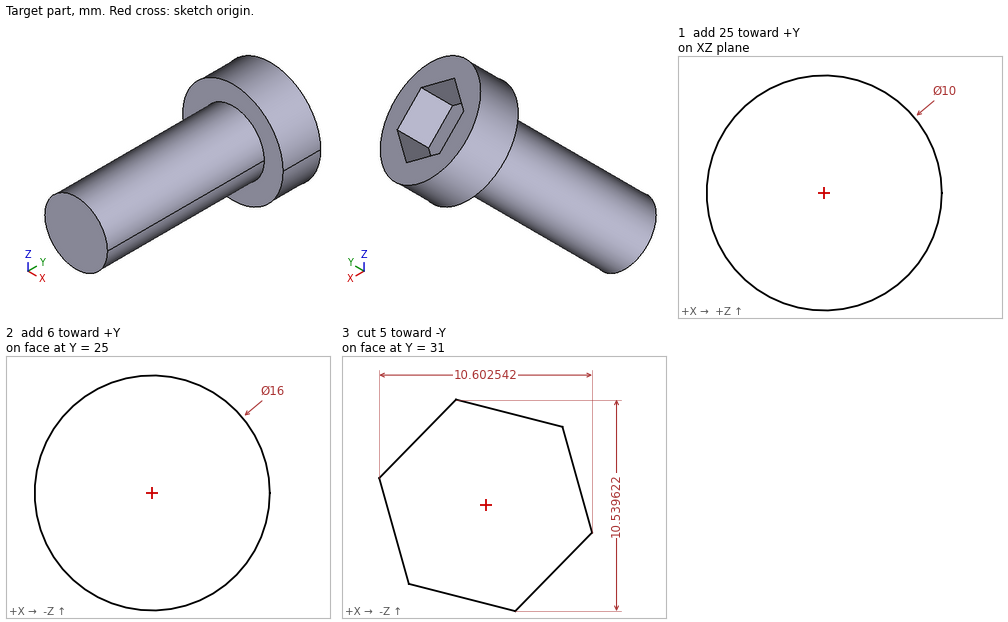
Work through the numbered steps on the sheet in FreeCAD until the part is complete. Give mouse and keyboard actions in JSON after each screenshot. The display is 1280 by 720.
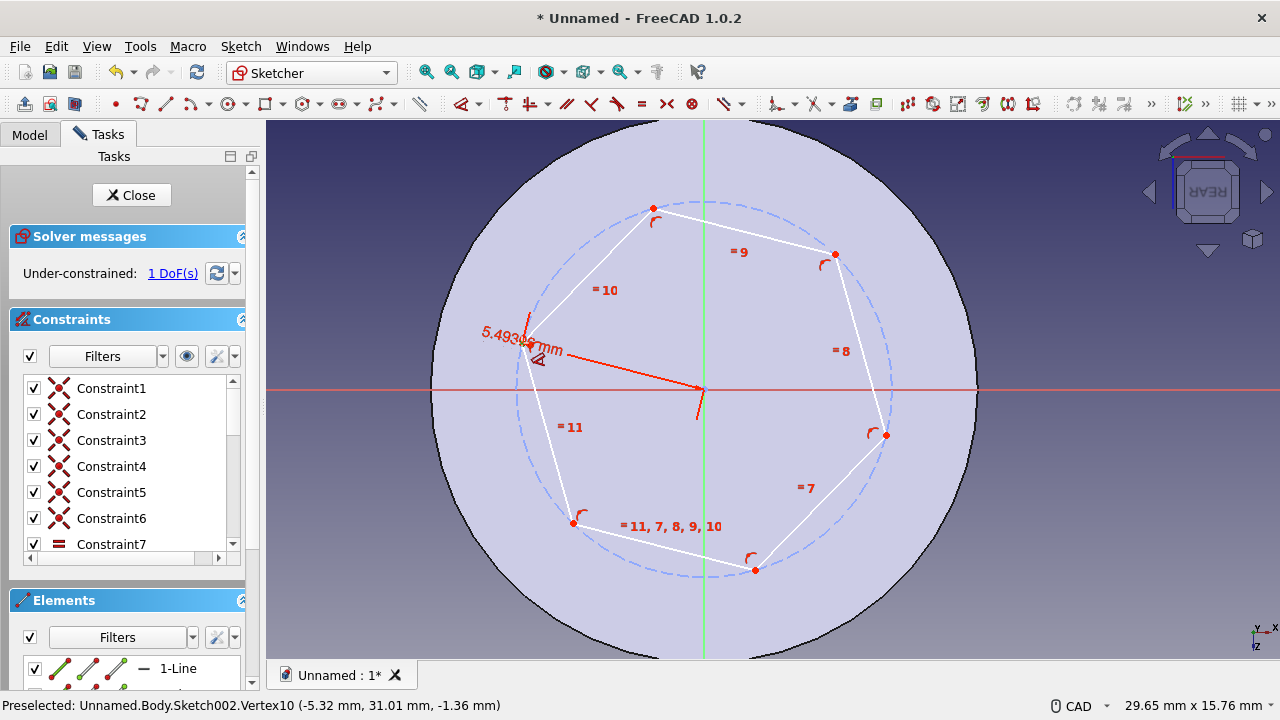
{"action": "left_click", "coordinate": [886, 436]}
{"action": "left_click", "coordinate": [620, 309]}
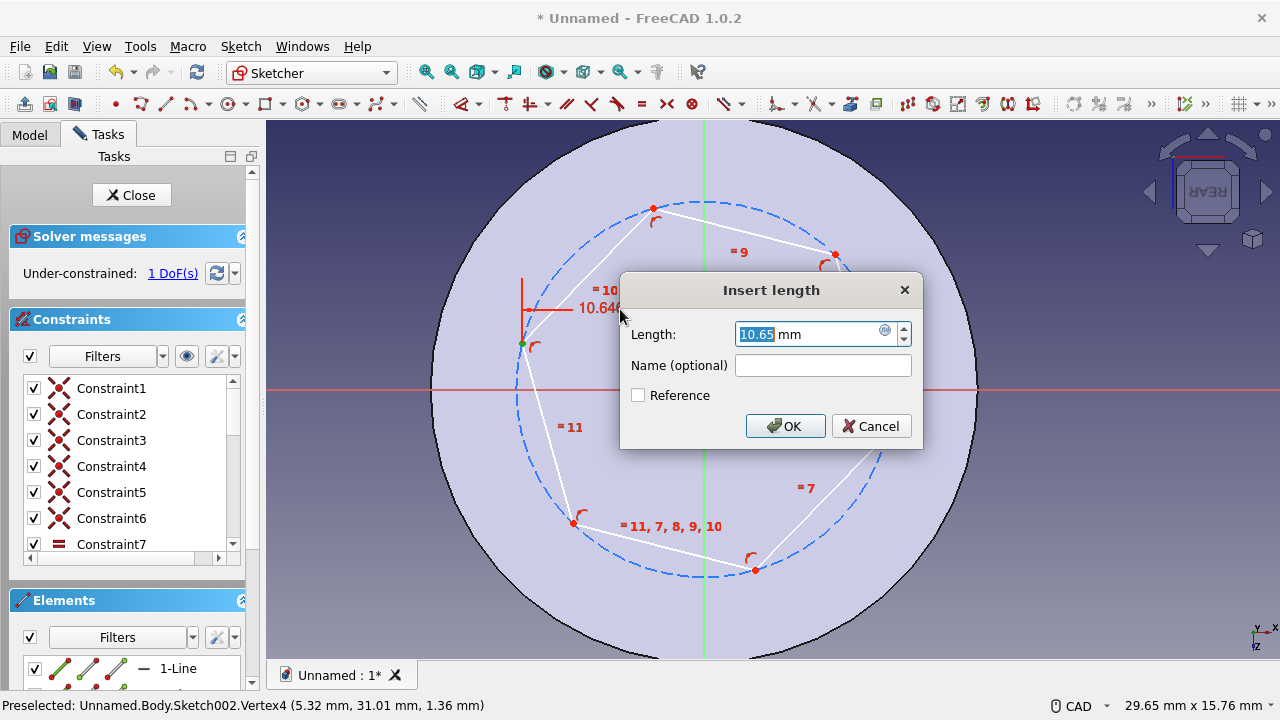
{"action": "type", "text": "10.602542"}
{"action": "key", "text": "Return"}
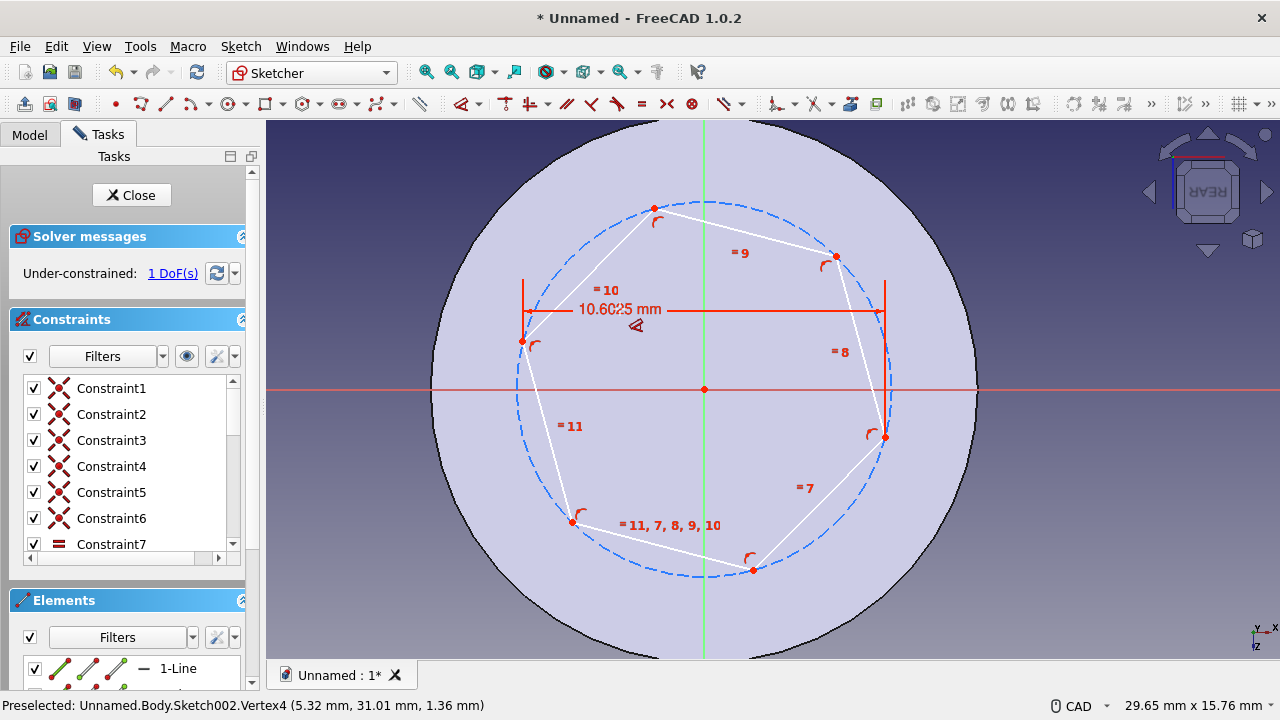
{"action": "left_click", "coordinate": [754, 570]}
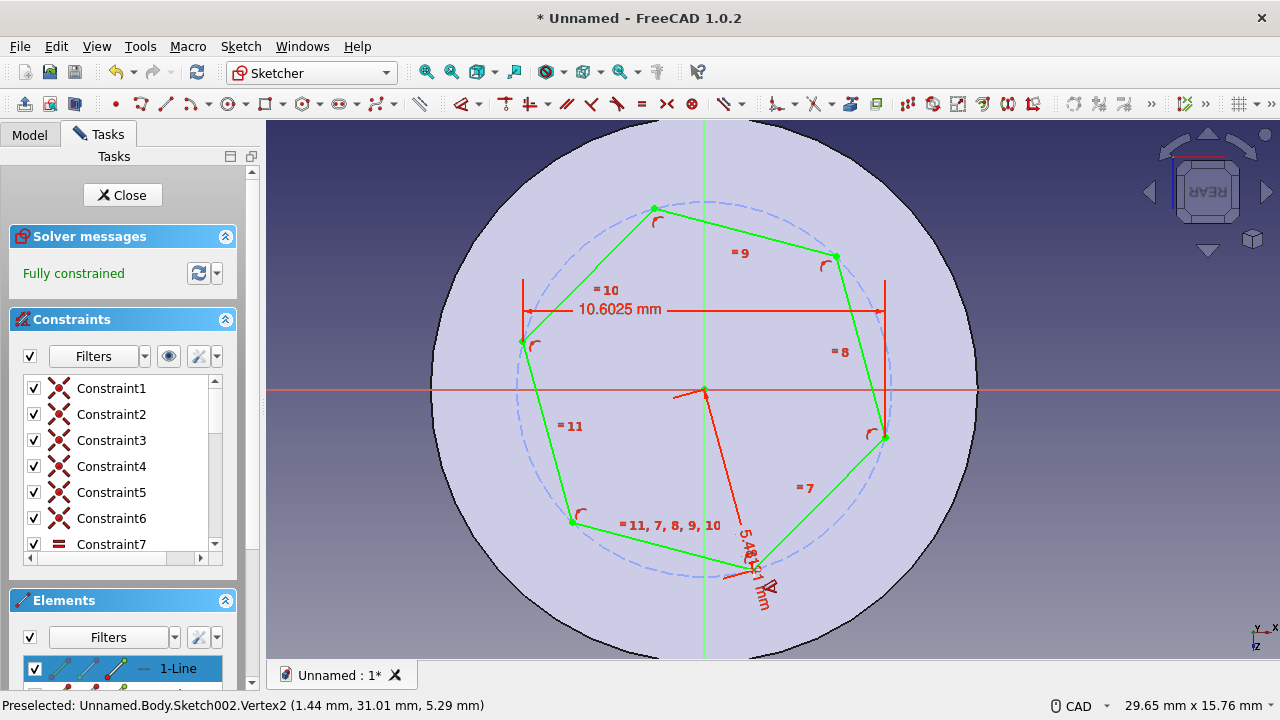
{"action": "left_click", "coordinate": [655, 209]}
{"action": "left_click", "coordinate": [788, 306]}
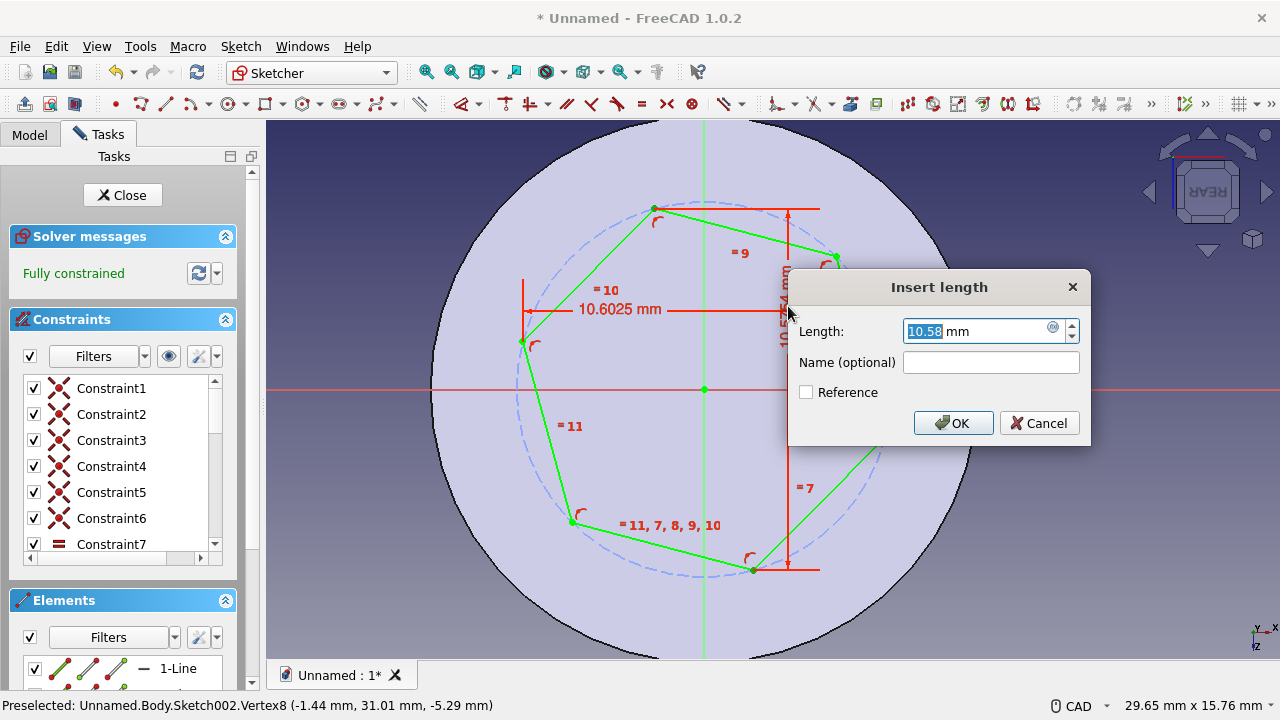
{"action": "type", "text": "10.539622"}
{"action": "key", "text": "Return"}
{"action": "key", "text": "Escape"}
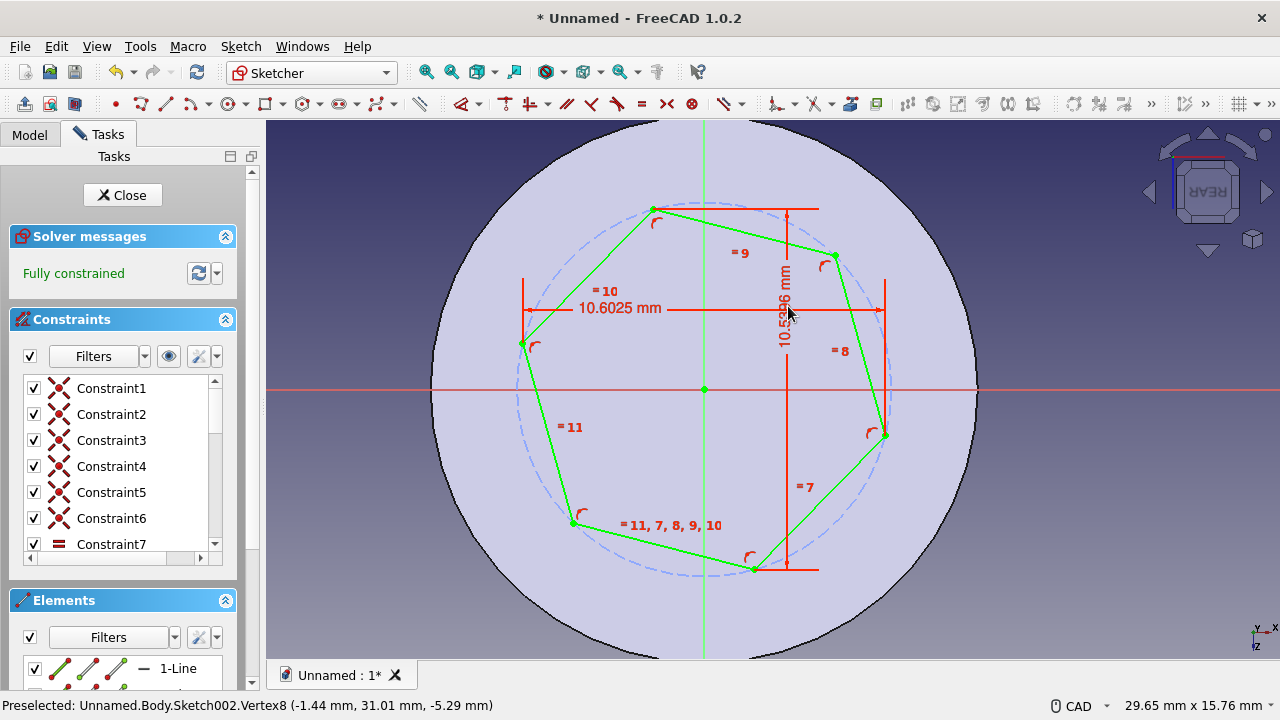
{"action": "left_click", "coordinate": [123, 195]}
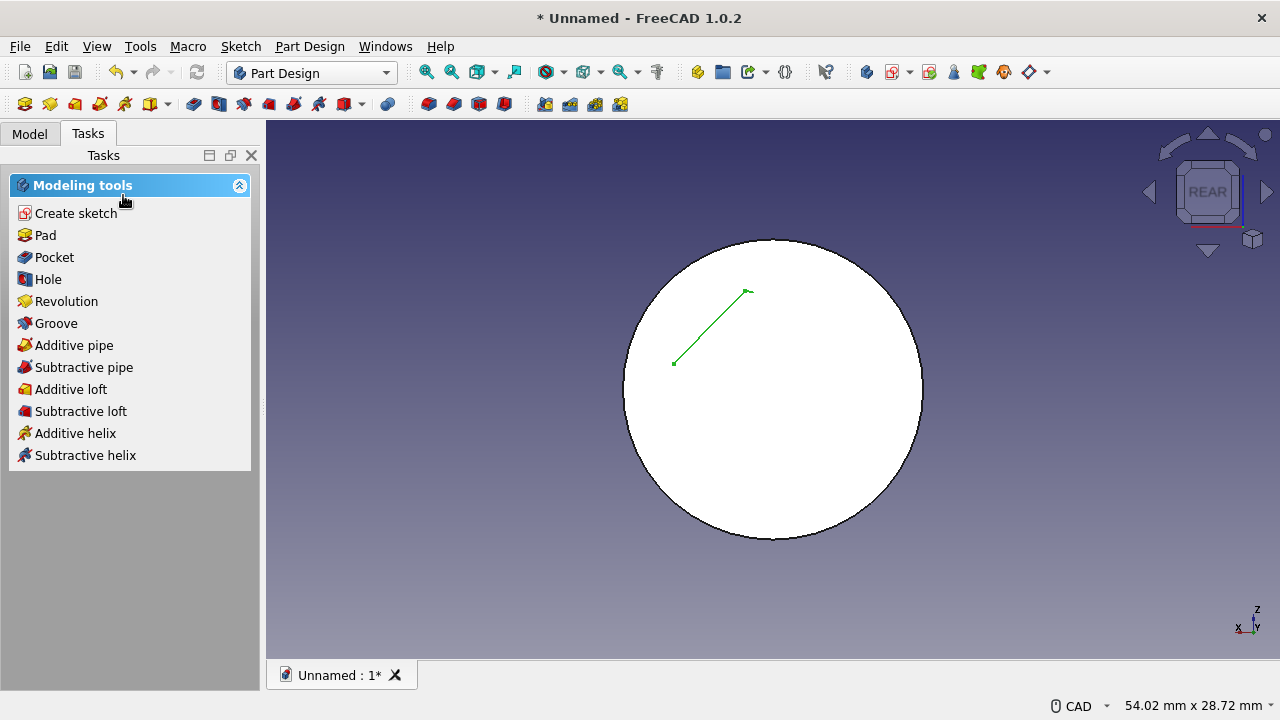
{"action": "left_click", "coordinate": [194, 104]}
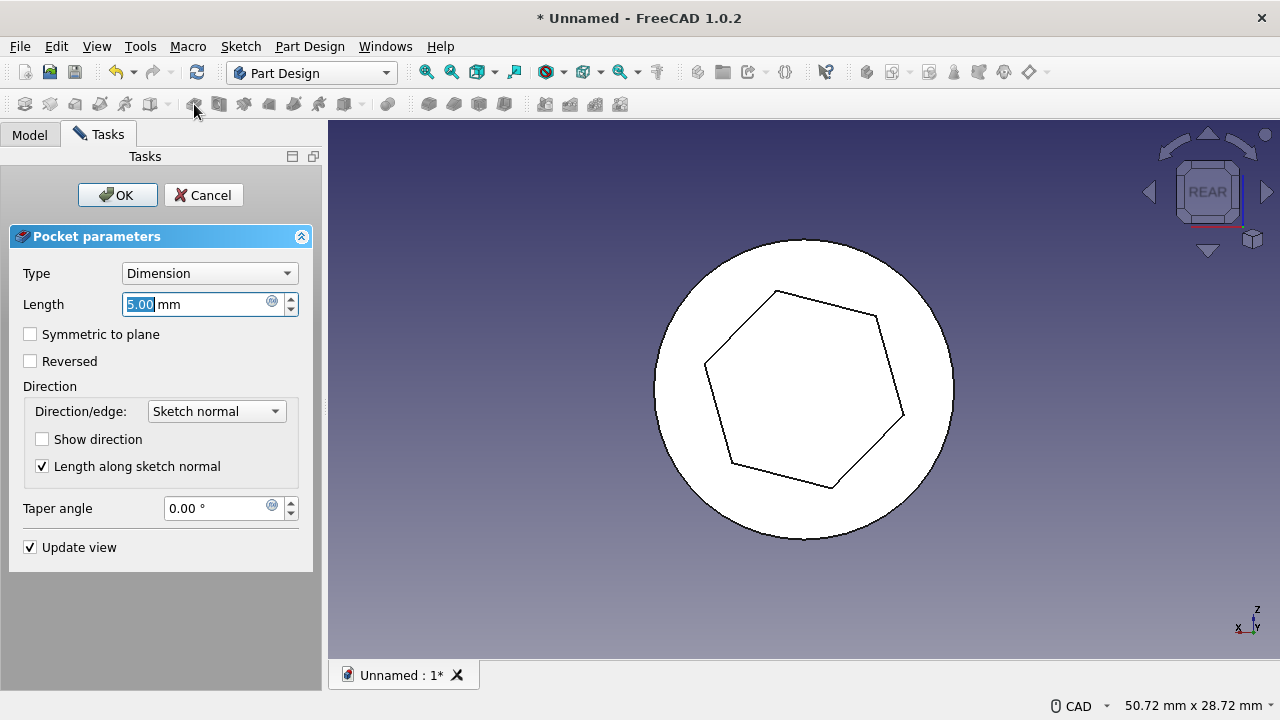
{"action": "type", "text": "5"}
{"action": "key", "text": "Tab"}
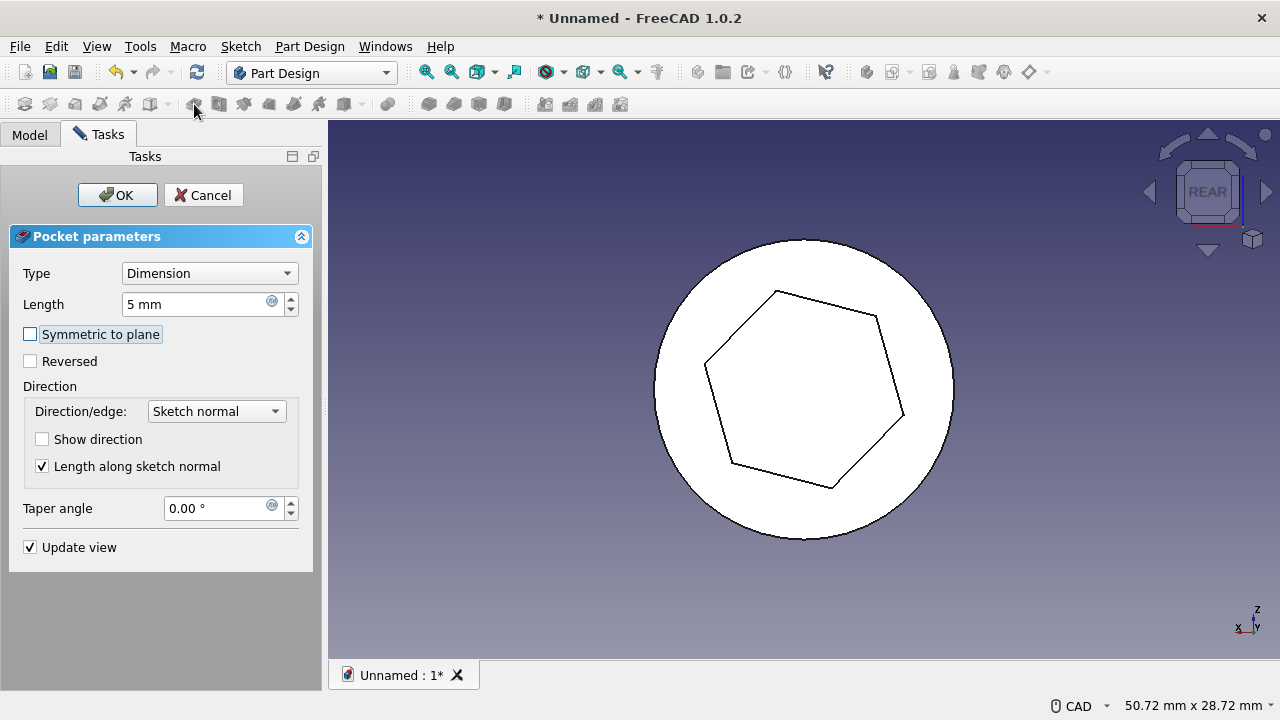
{"action": "left_click", "coordinate": [118, 195]}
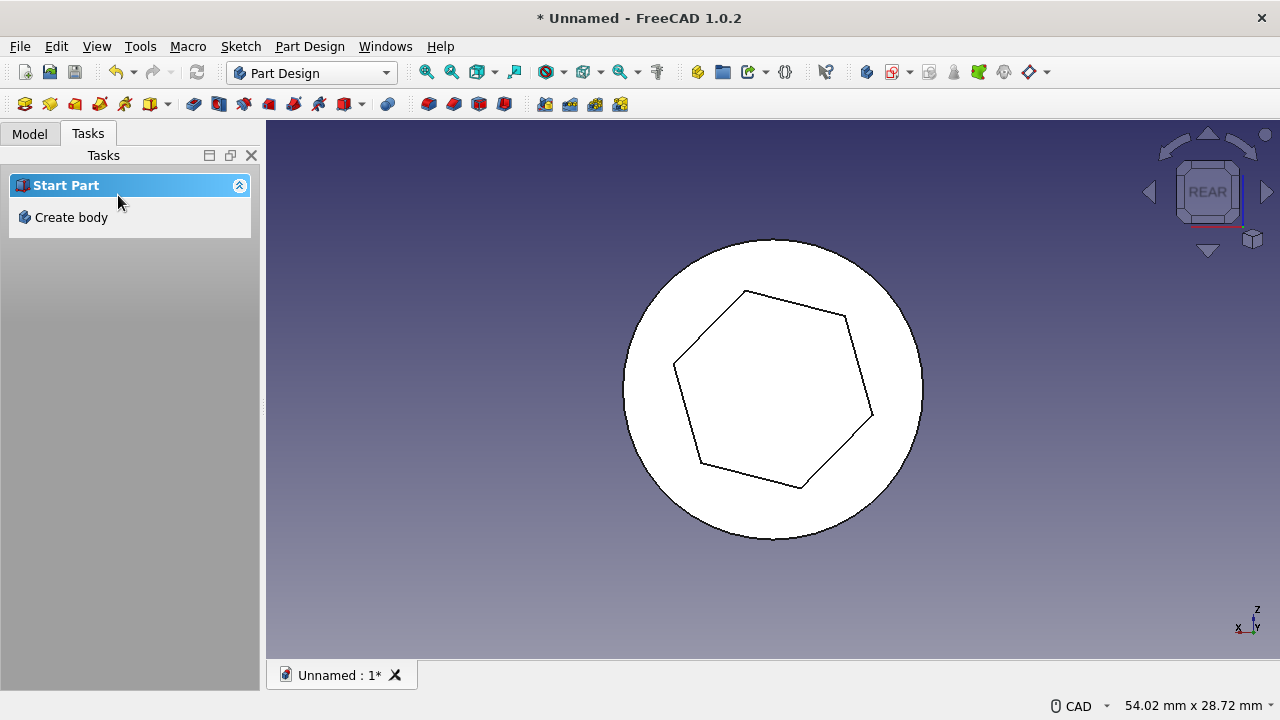
{"action": "key", "text": "0"}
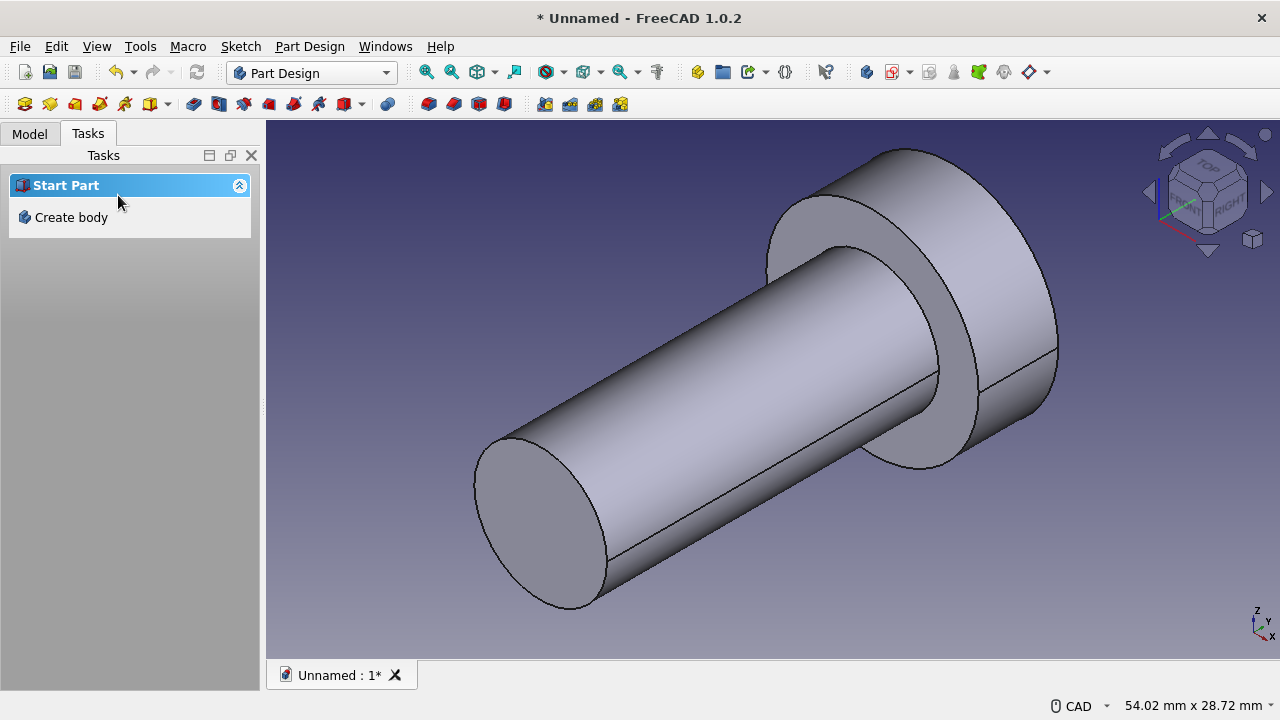
{"action": "key", "text": "v f"}